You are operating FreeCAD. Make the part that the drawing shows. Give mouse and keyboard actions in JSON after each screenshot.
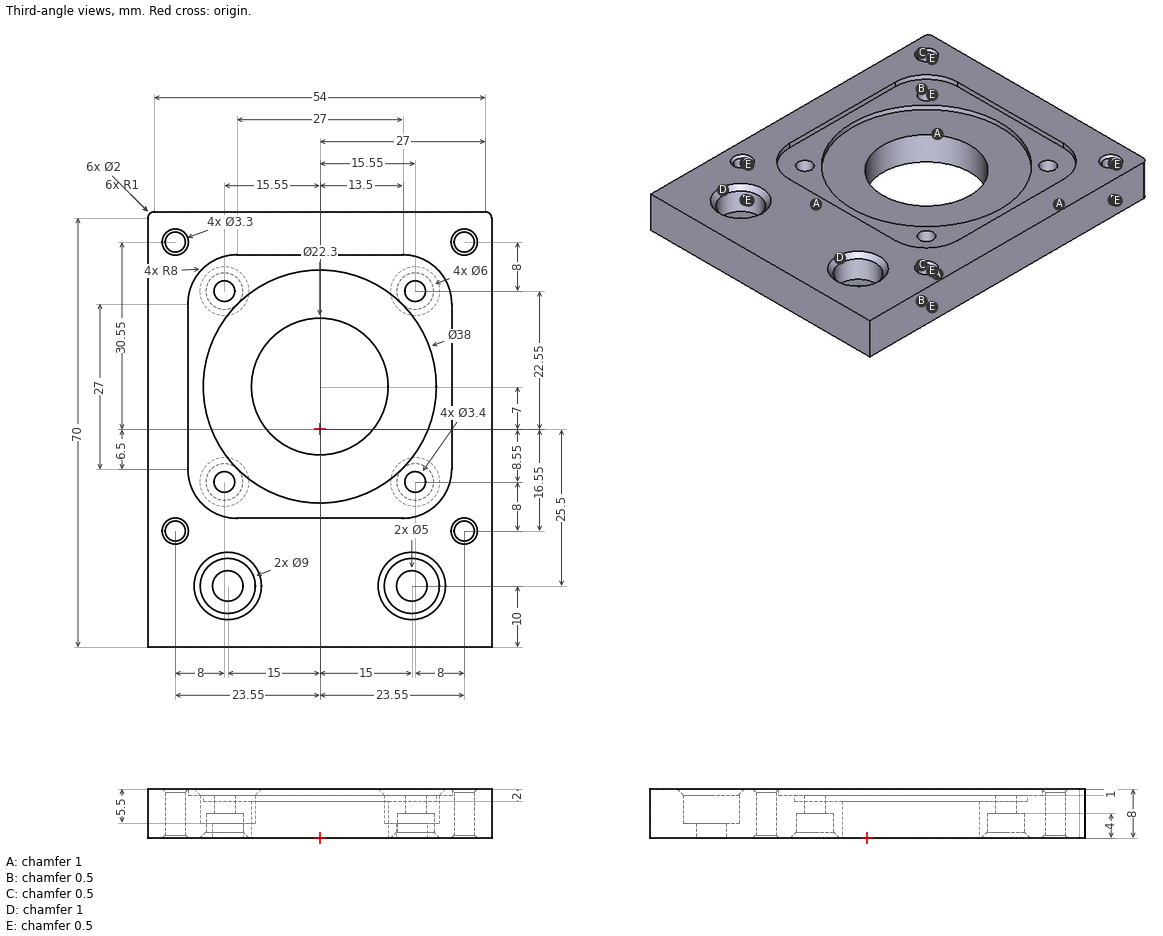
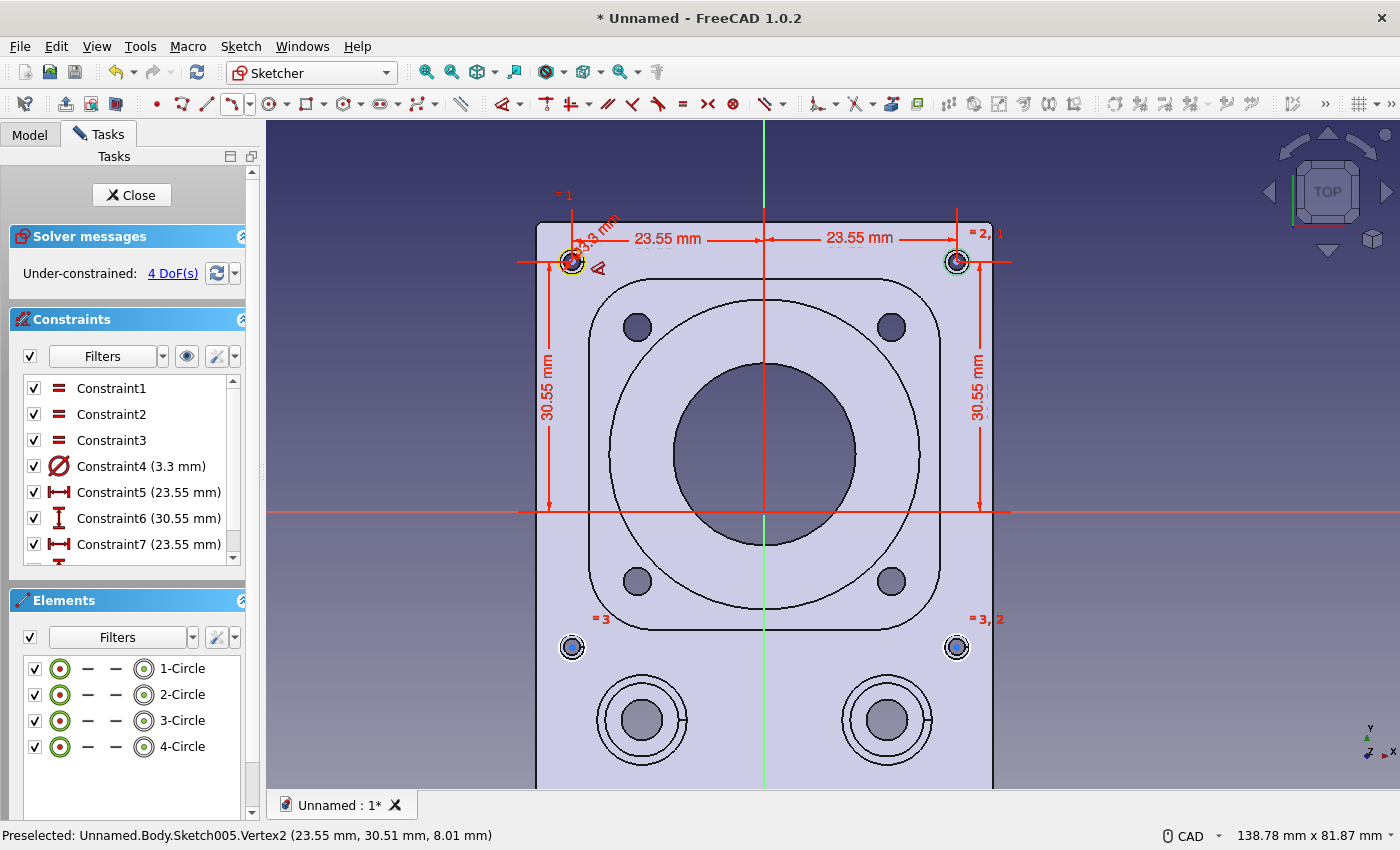
{"action": "left_click", "coordinate": [957, 648]}
{"action": "left_click", "coordinate": [861, 682]}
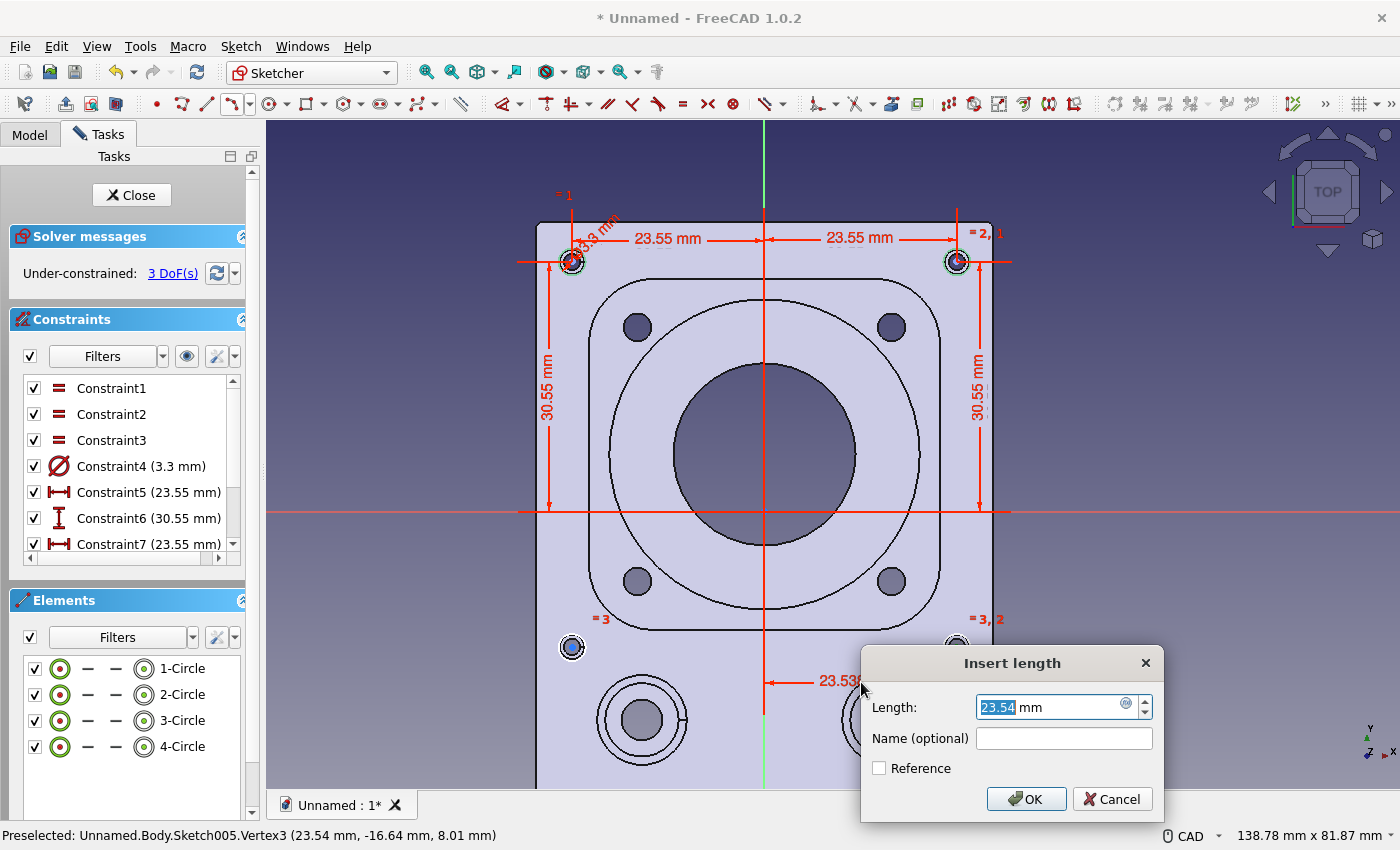
{"action": "type", "text": "23.55"}
{"action": "key", "text": "Return"}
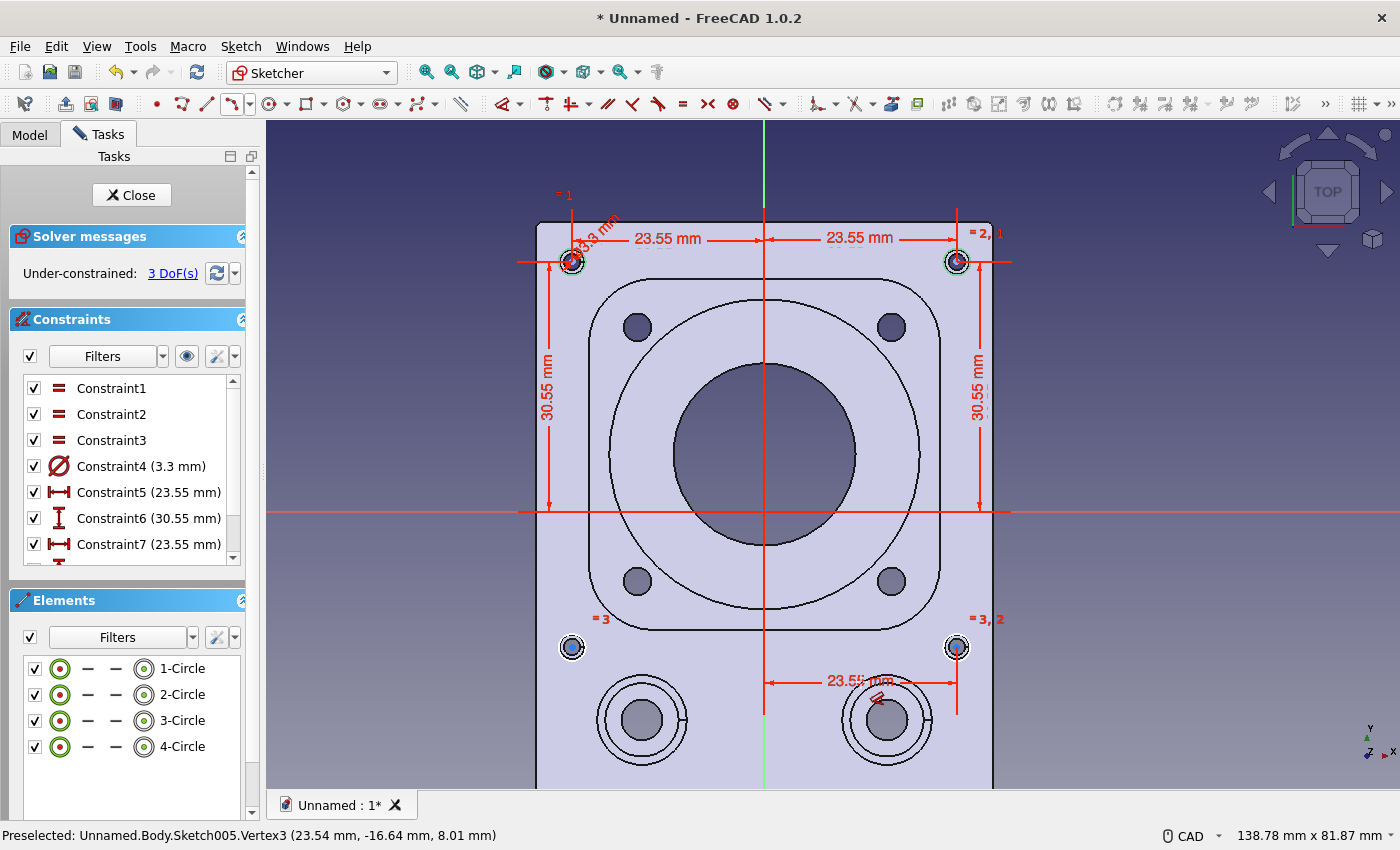
{"action": "left_click", "coordinate": [957, 648]}
{"action": "left_click", "coordinate": [991, 580]}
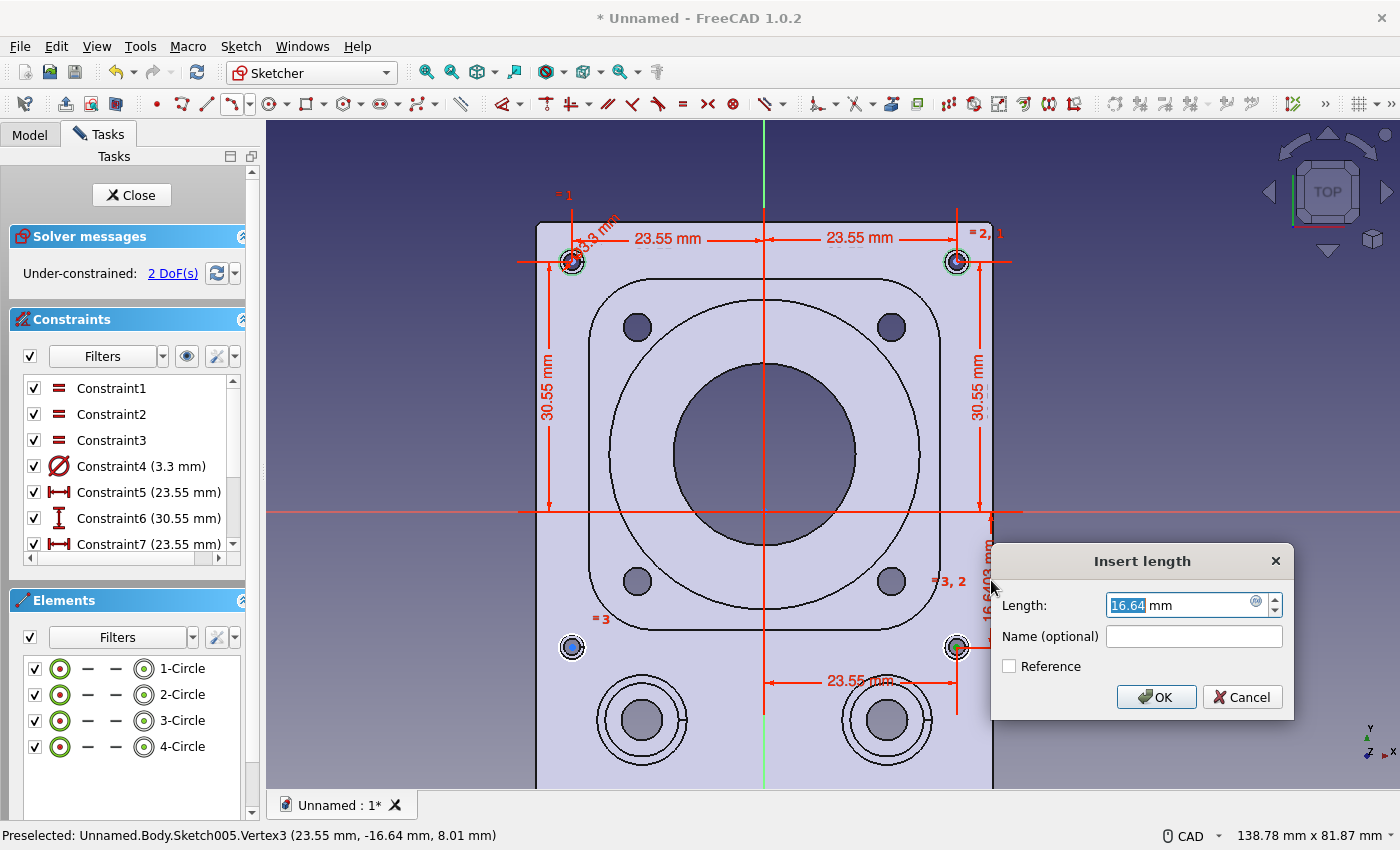
{"action": "type", "text": "16.55"}
{"action": "key", "text": "Return"}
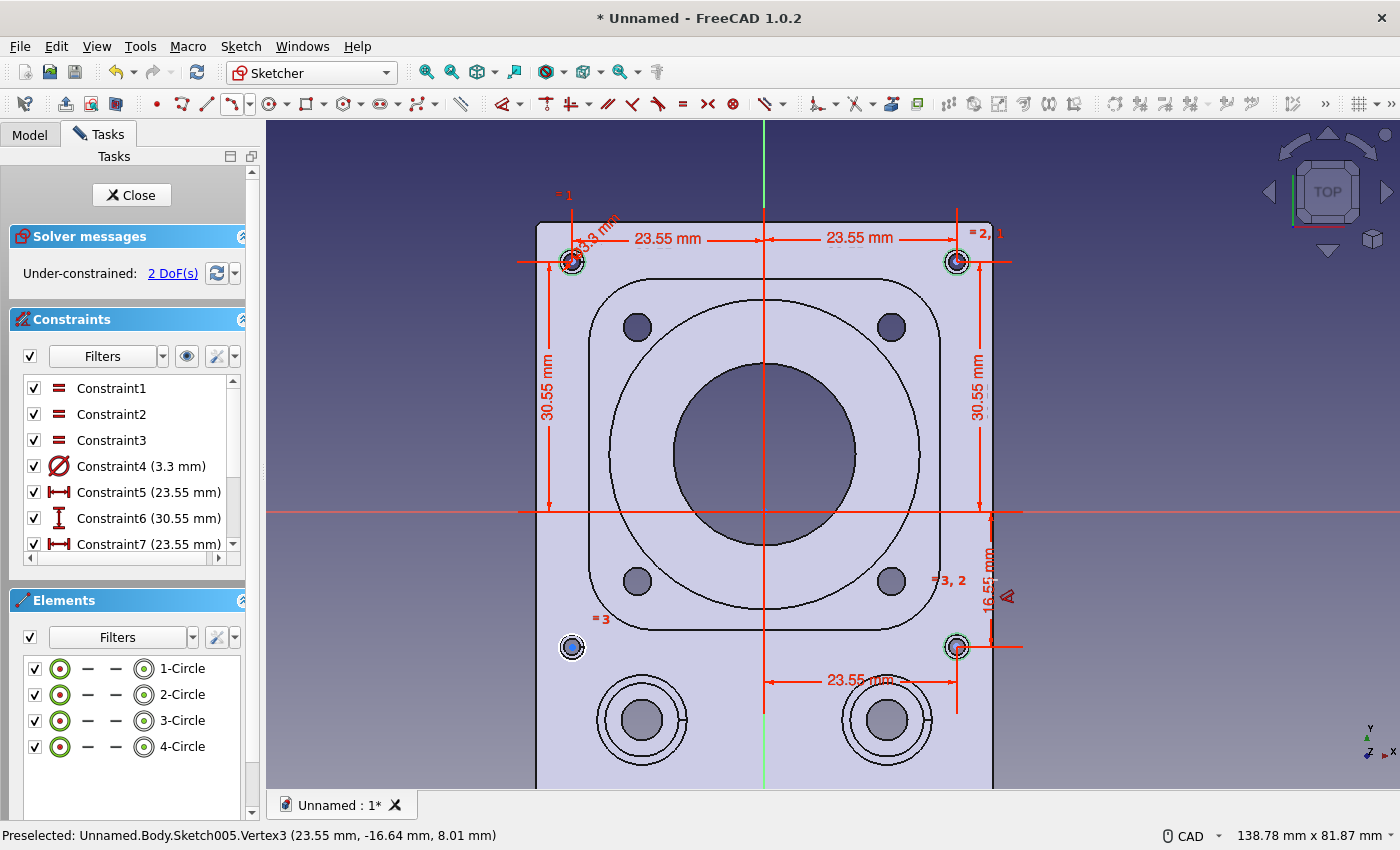
{"action": "left_click", "coordinate": [572, 648]}
{"action": "left_click", "coordinate": [668, 682]}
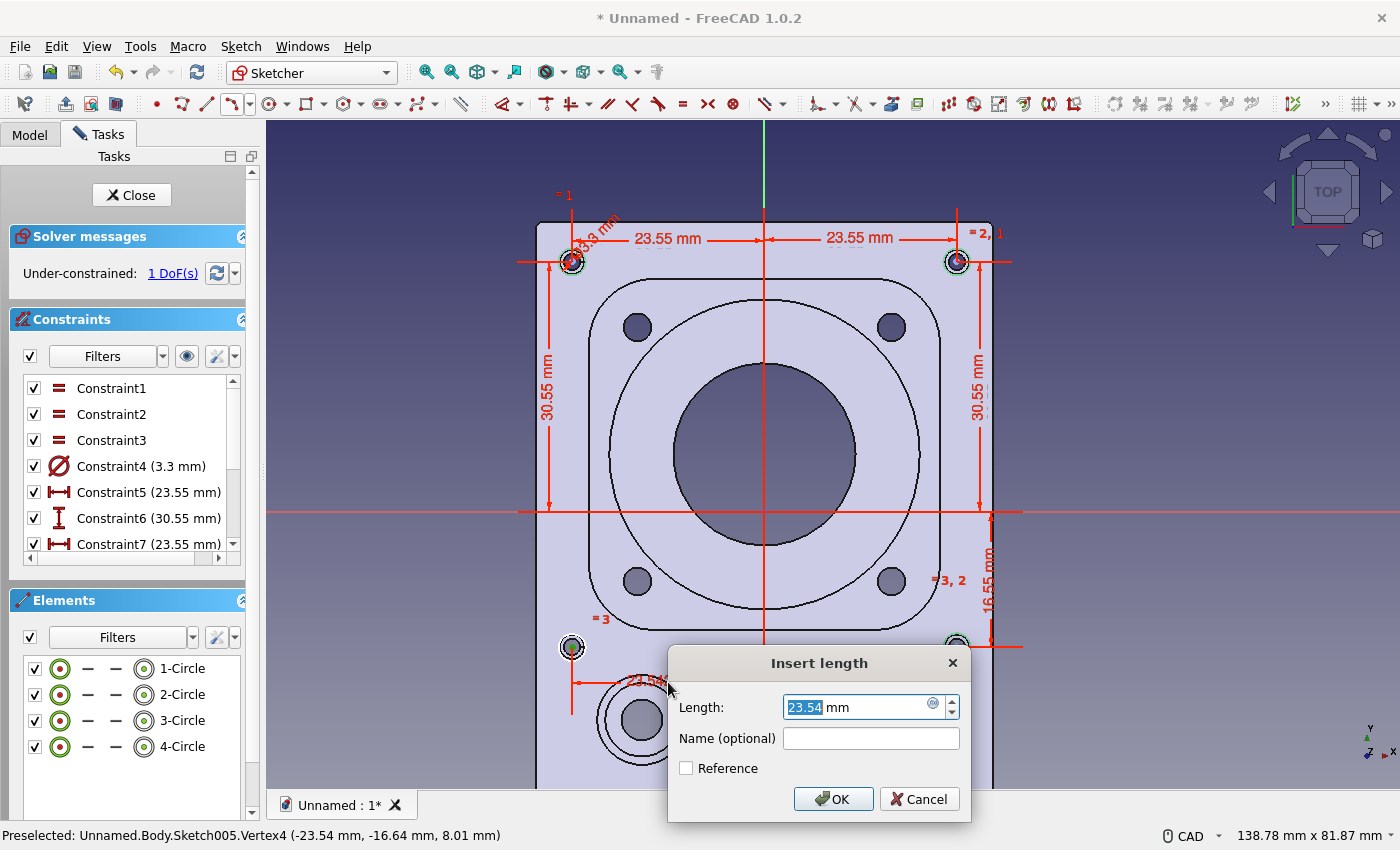
{"action": "type", "text": "23.55"}
{"action": "key", "text": "Return"}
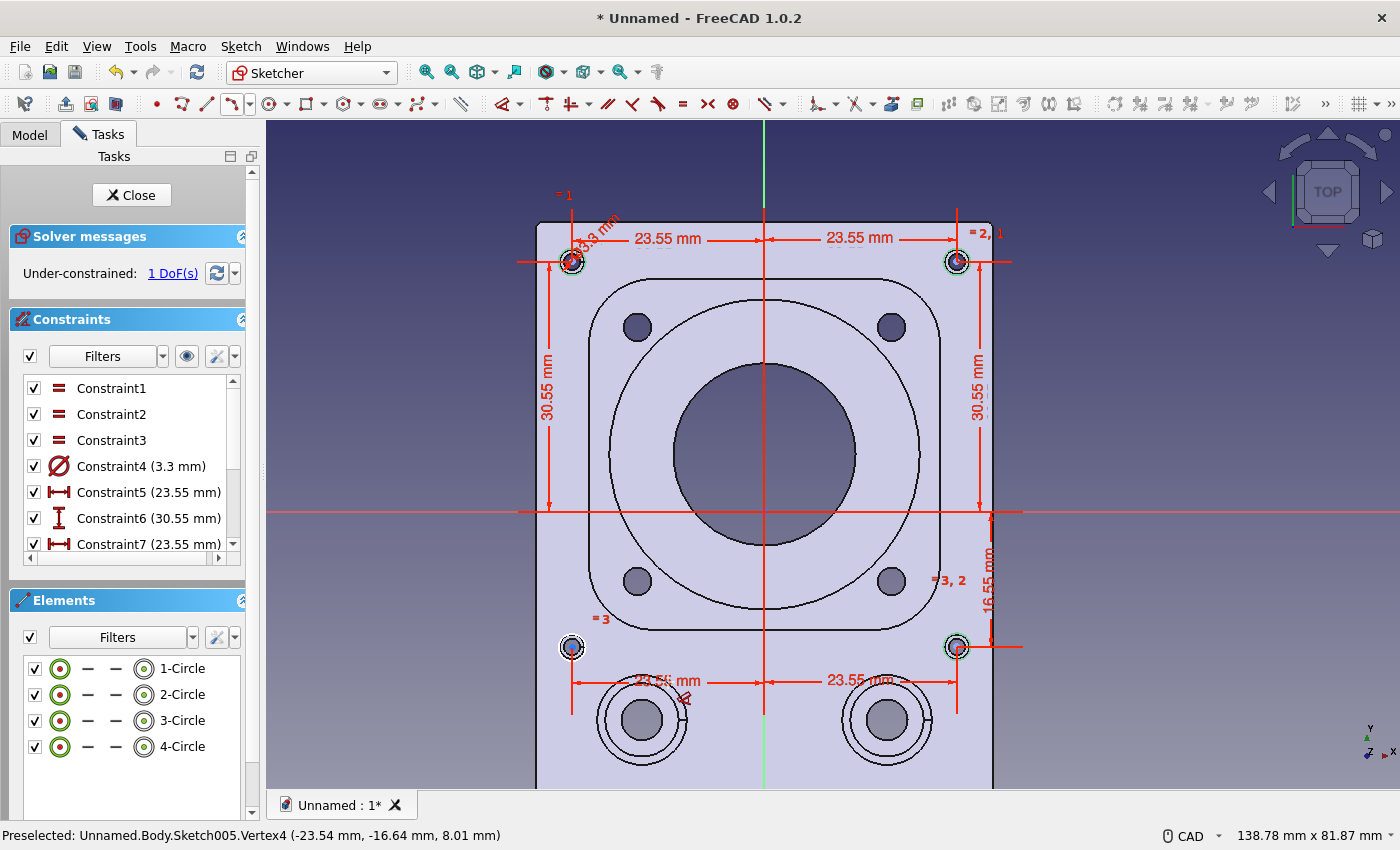
{"action": "left_click", "coordinate": [572, 648]}
{"action": "left_click", "coordinate": [538, 580]}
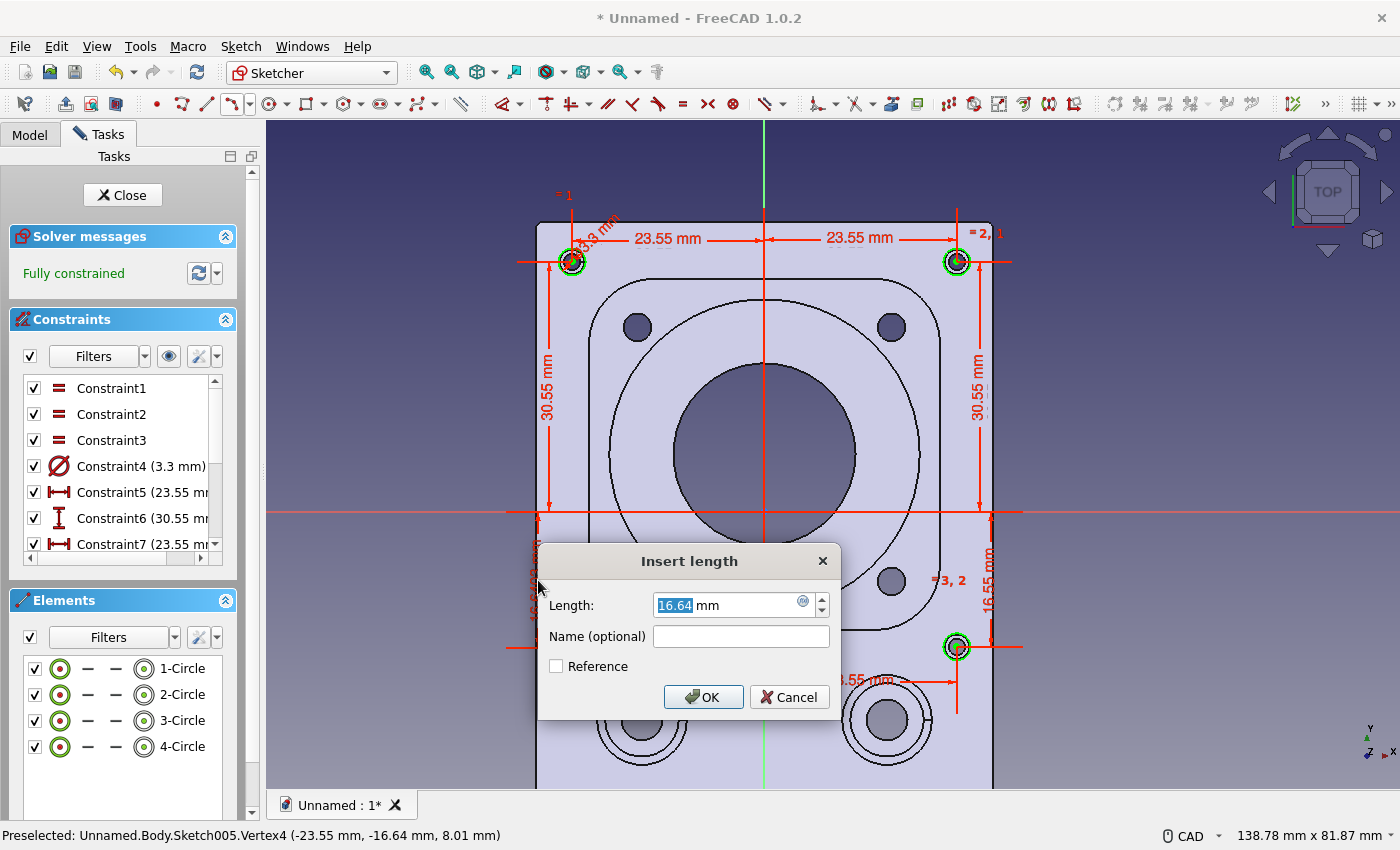
{"action": "type", "text": "16.55"}
{"action": "key", "text": "Return"}
{"action": "key", "text": "Escape"}